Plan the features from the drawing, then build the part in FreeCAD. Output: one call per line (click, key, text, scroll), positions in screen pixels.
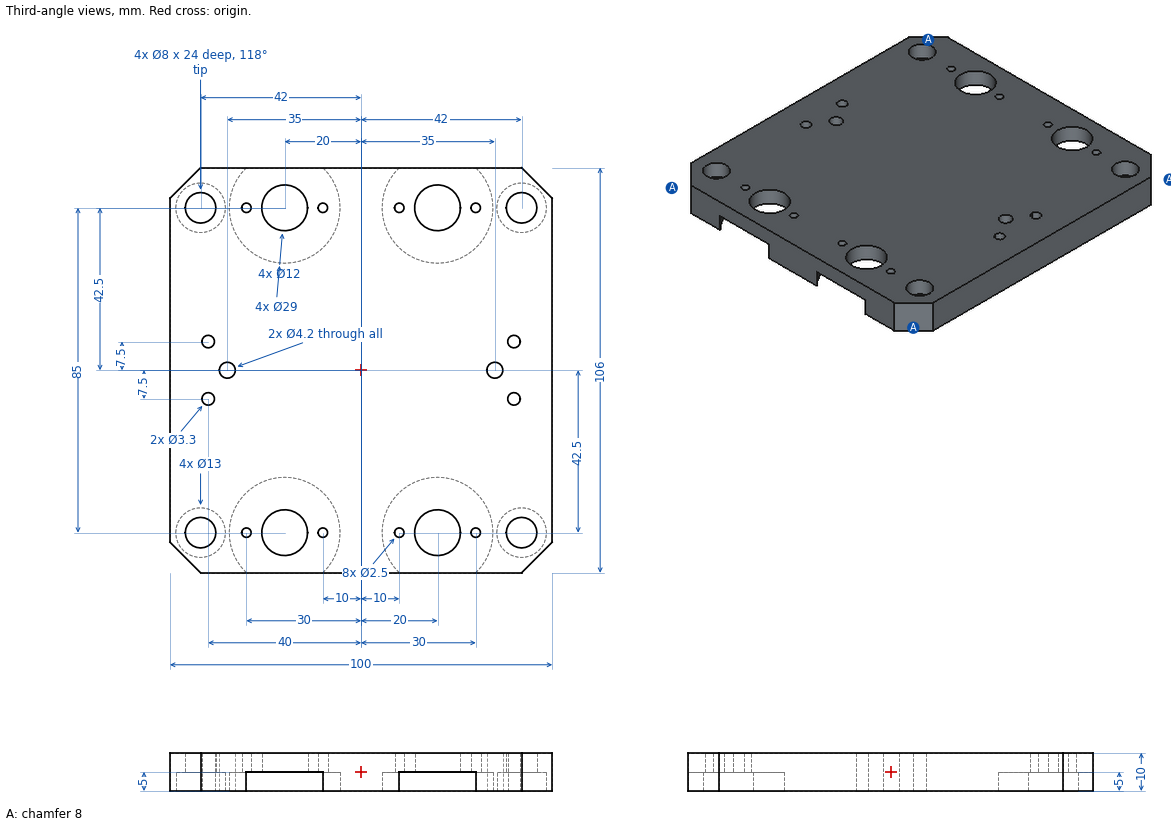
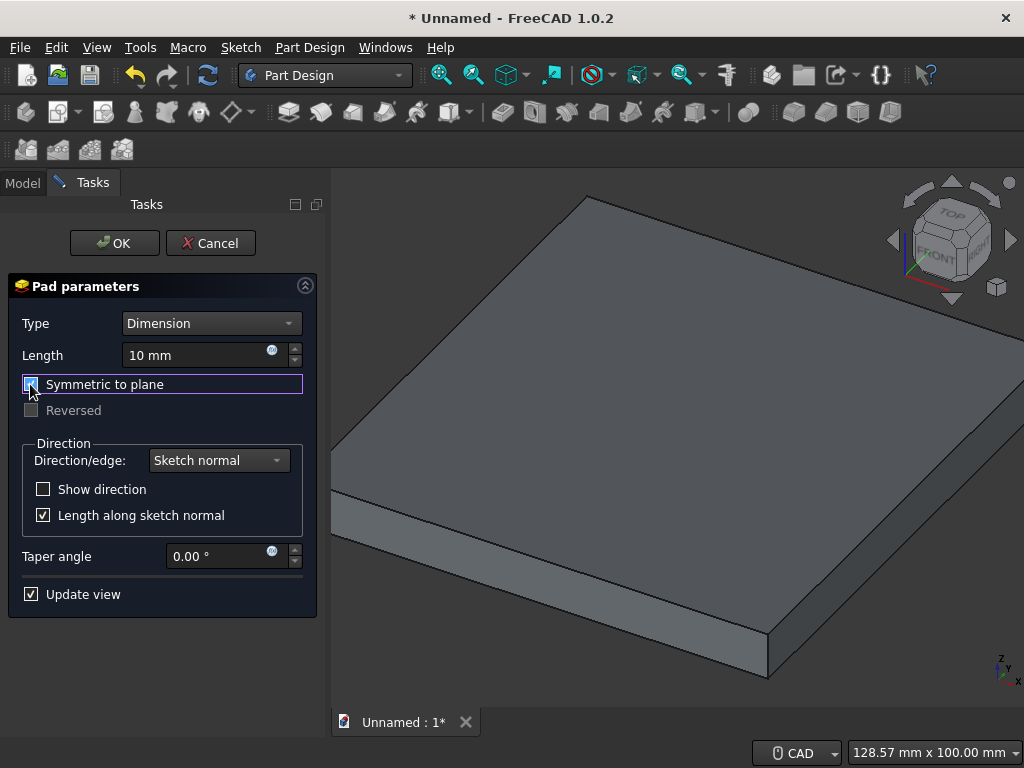
click(115, 243)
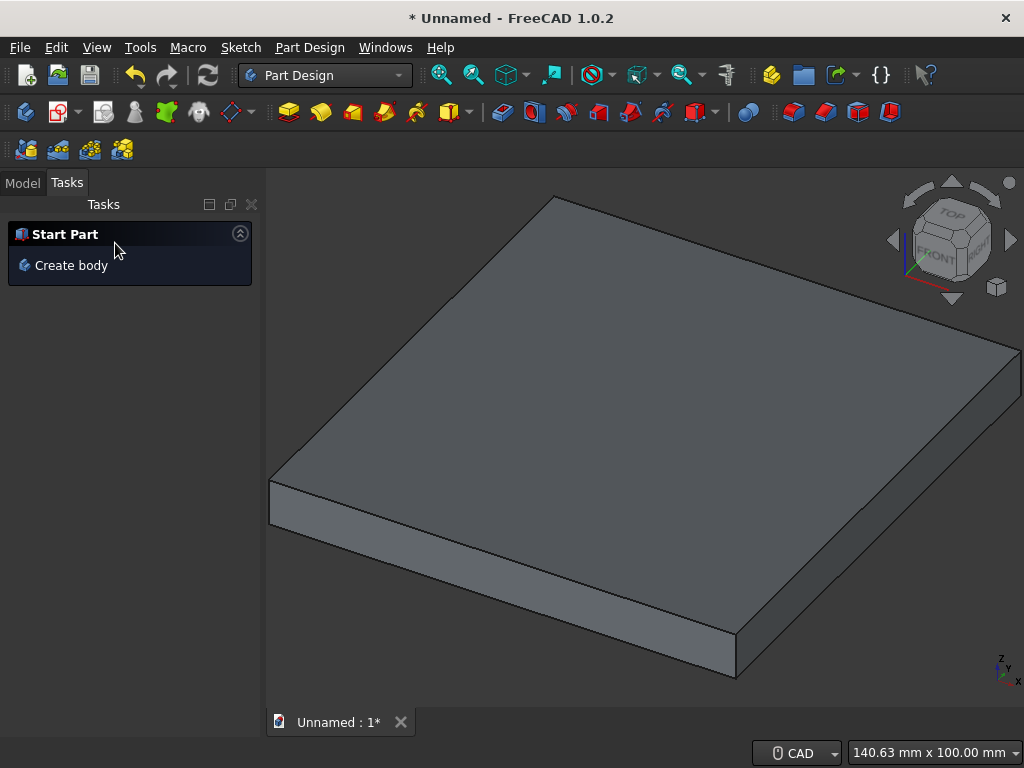
click(645, 414)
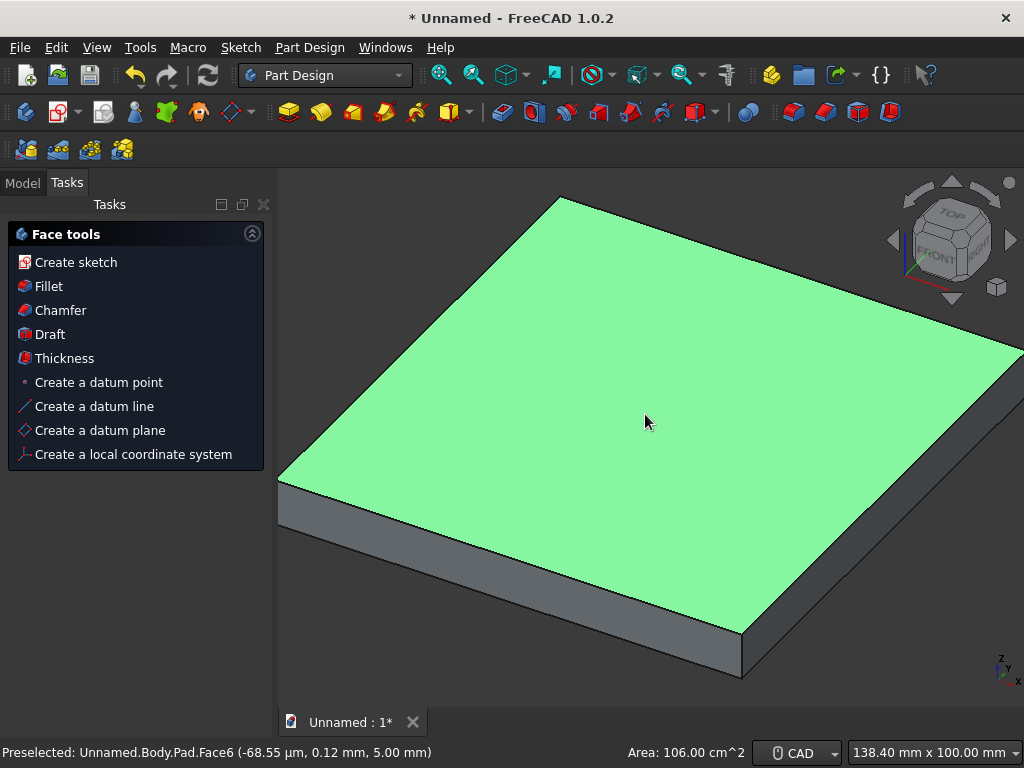
click(58, 112)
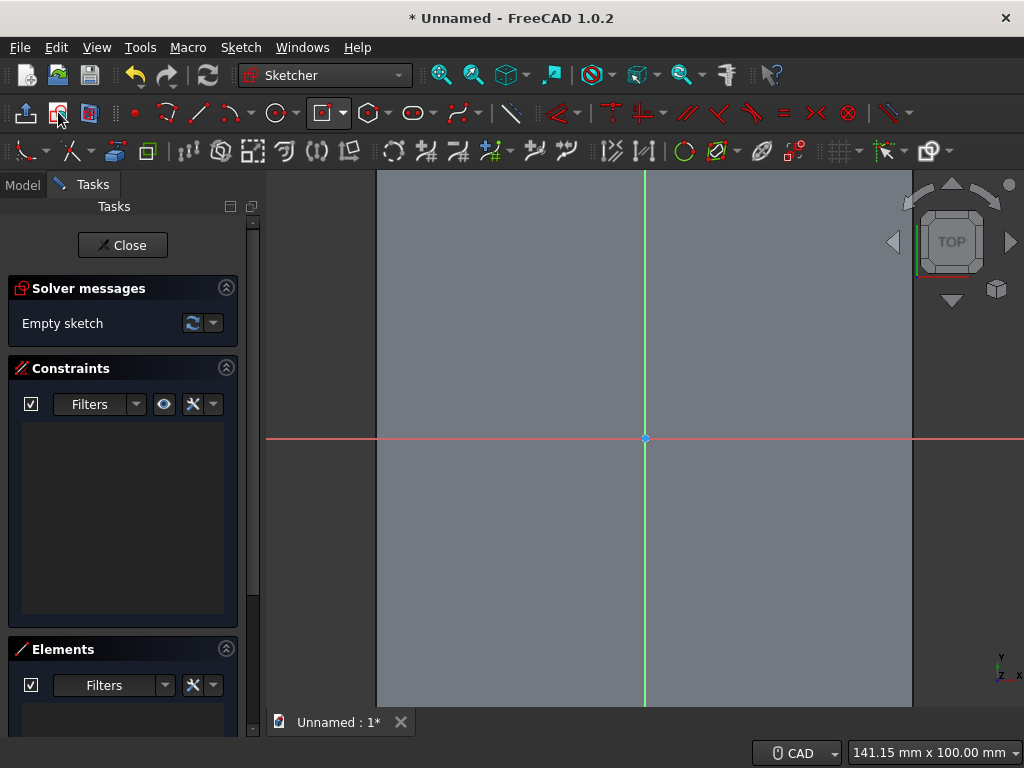
scroll(294, 439, down, 1)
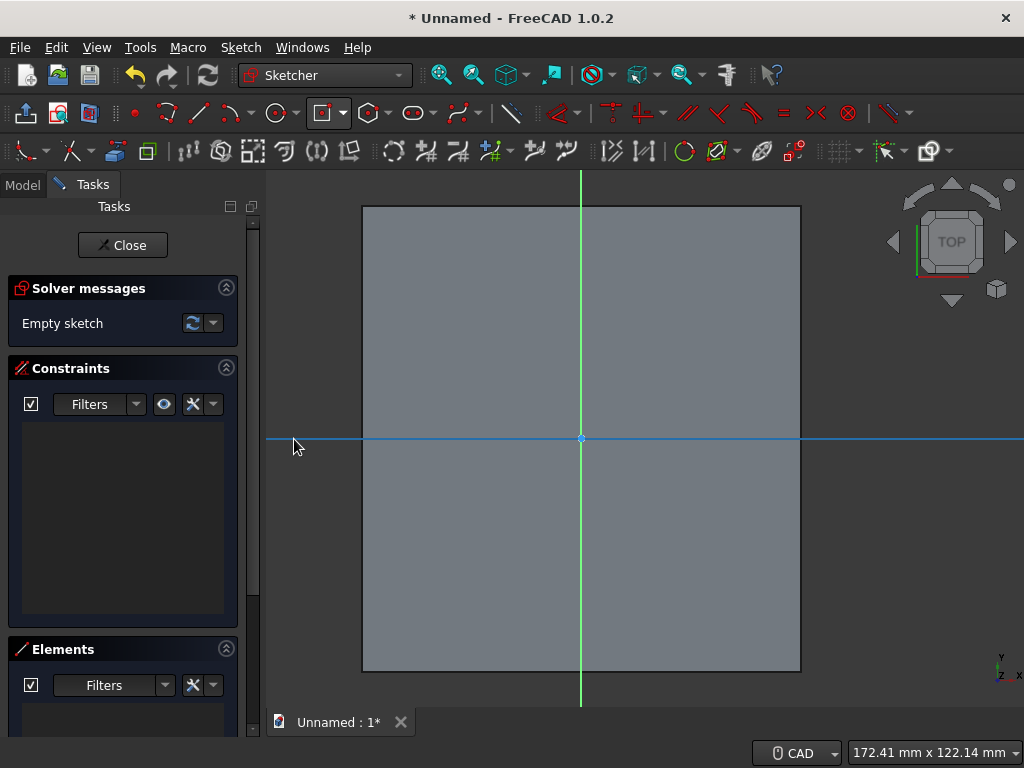
click(276, 114)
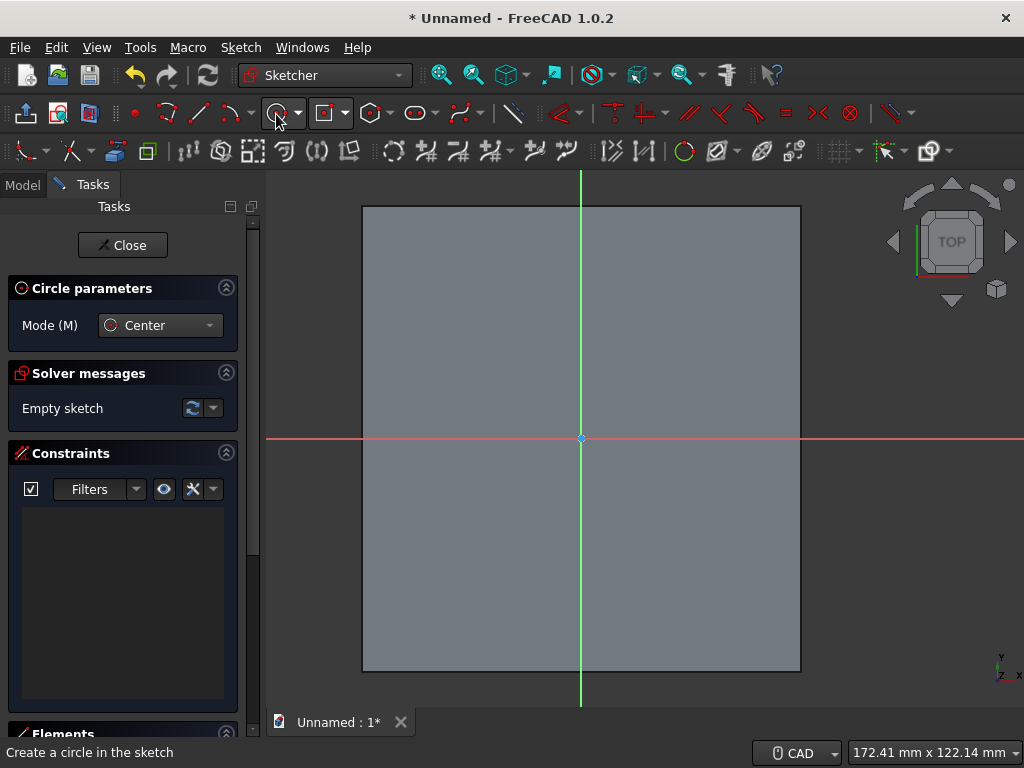
scroll(428, 439, up, 5)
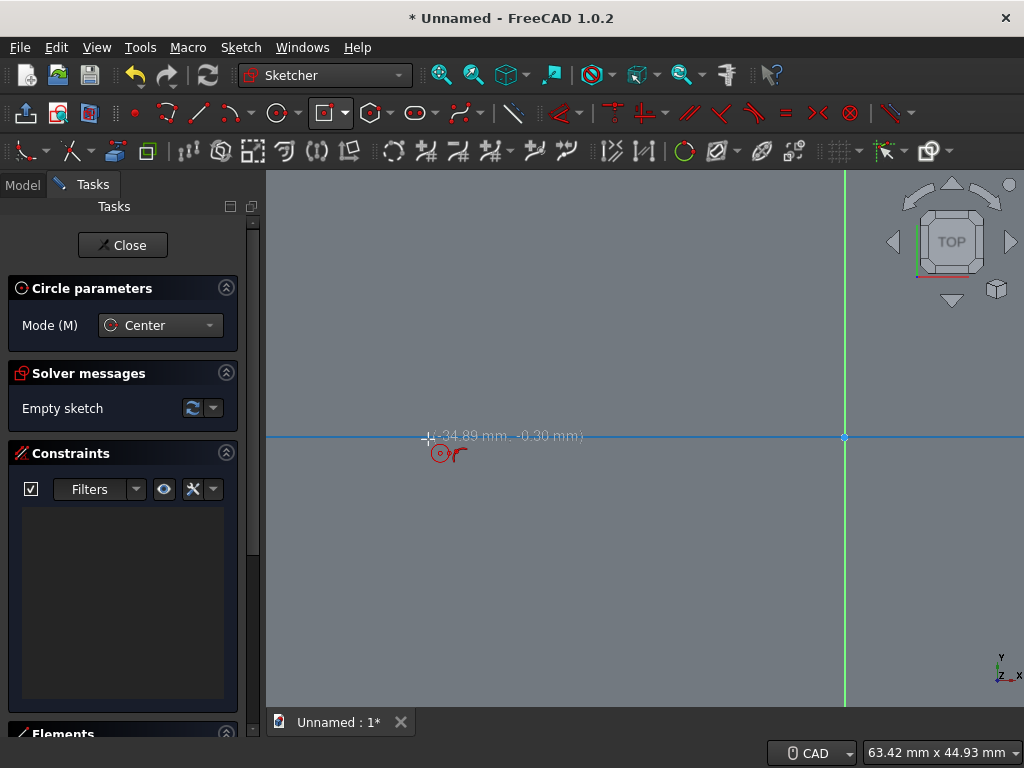
click(426, 437)
move(444, 420)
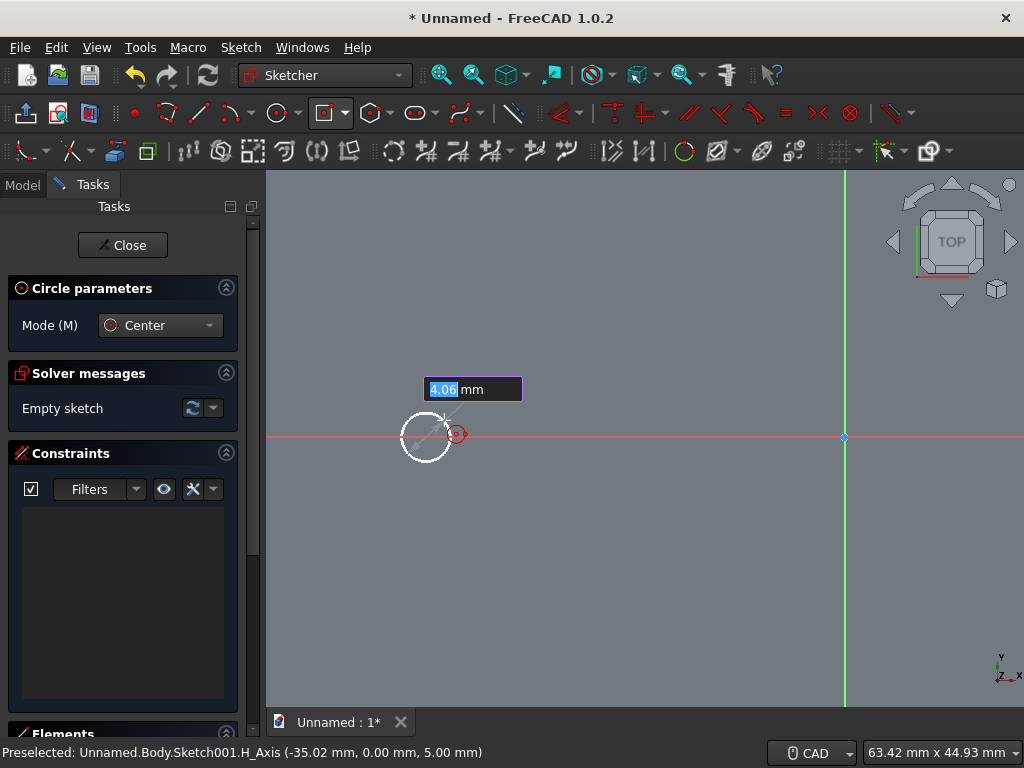
text(4.2)
key(Return)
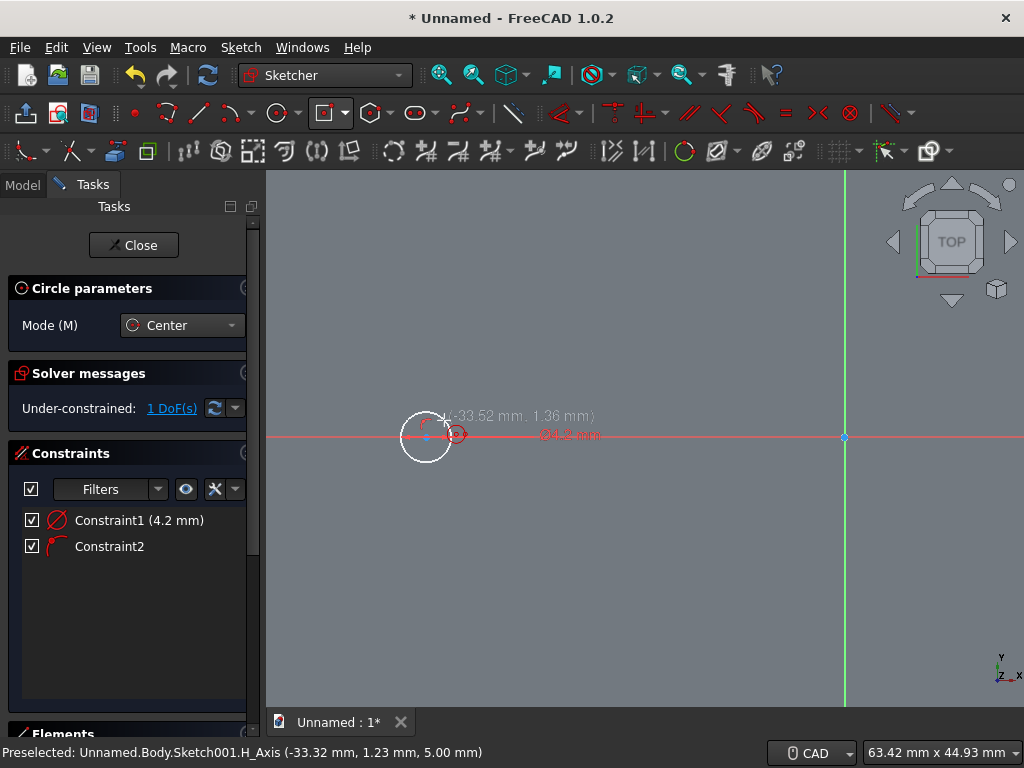
scroll(358, 440, down, 4)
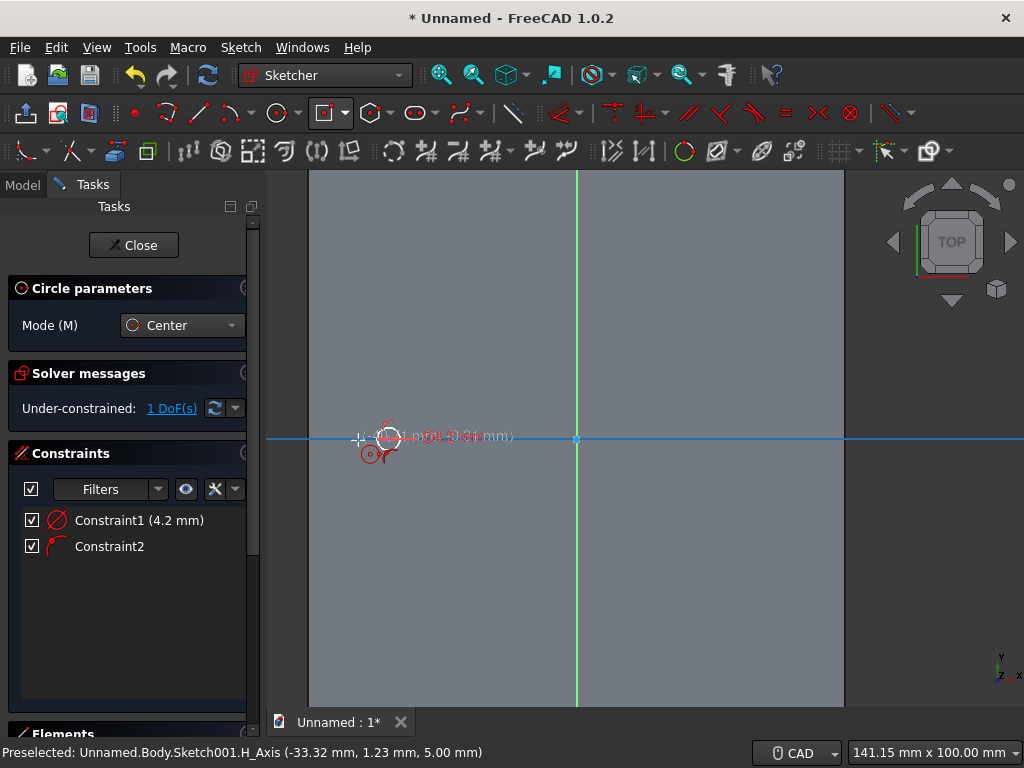
scroll(765, 439, up, 4)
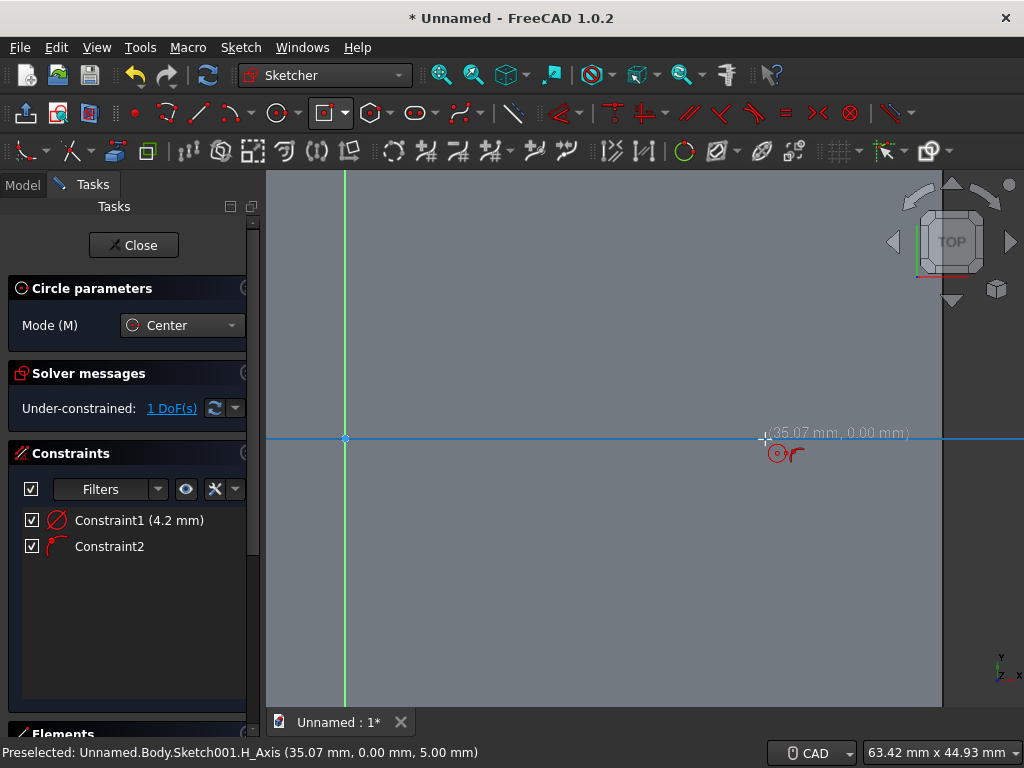
click(763, 438)
move(781, 421)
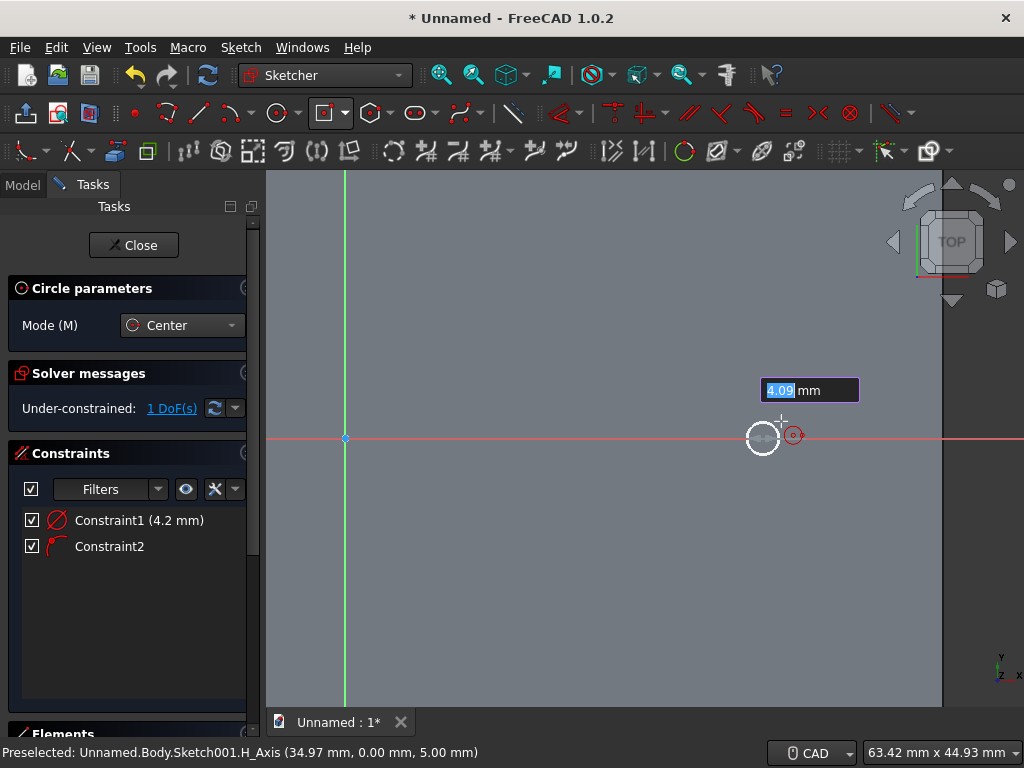
text(4.2)
key(Return)
key(Escape)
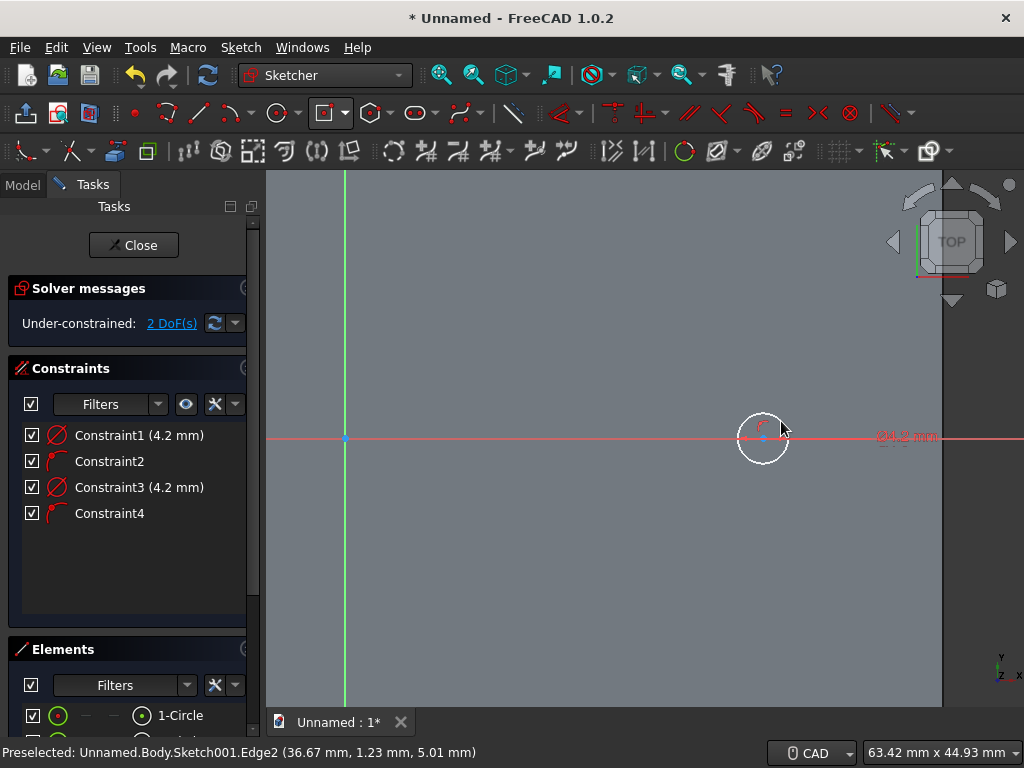
scroll(765, 439, down, 4)